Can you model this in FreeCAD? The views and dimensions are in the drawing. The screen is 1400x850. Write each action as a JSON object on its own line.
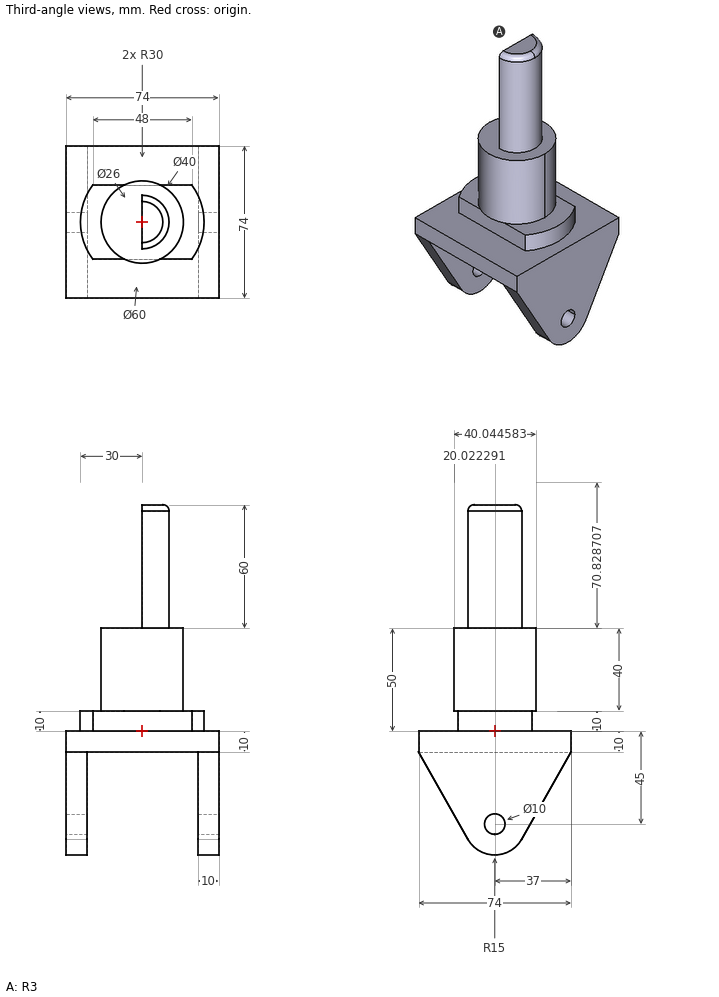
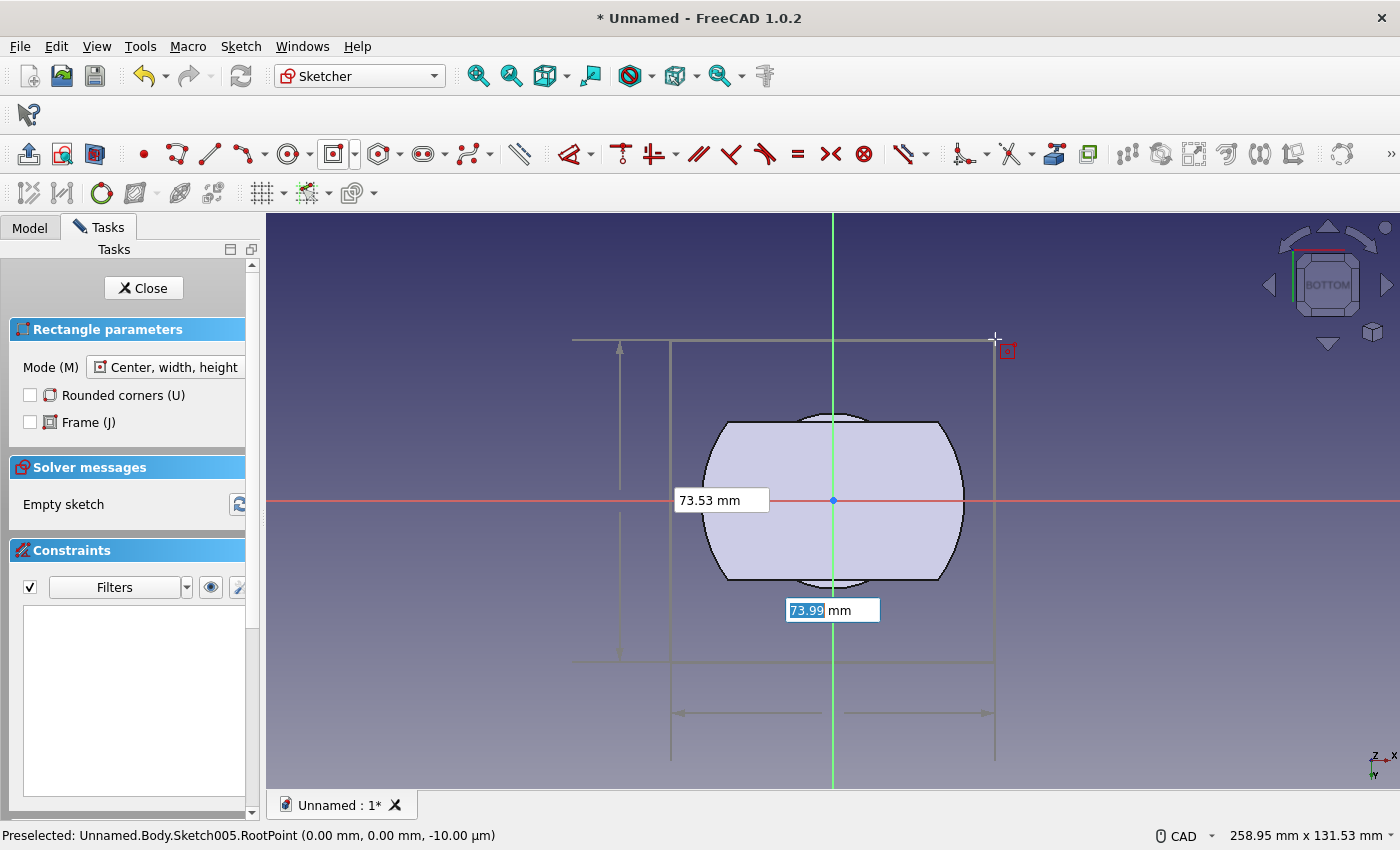
{"action": "type", "text": "74"}
{"action": "key", "text": "Tab"}
{"action": "type", "text": "74"}
{"action": "key", "text": "Return"}
{"action": "key", "text": "Escape"}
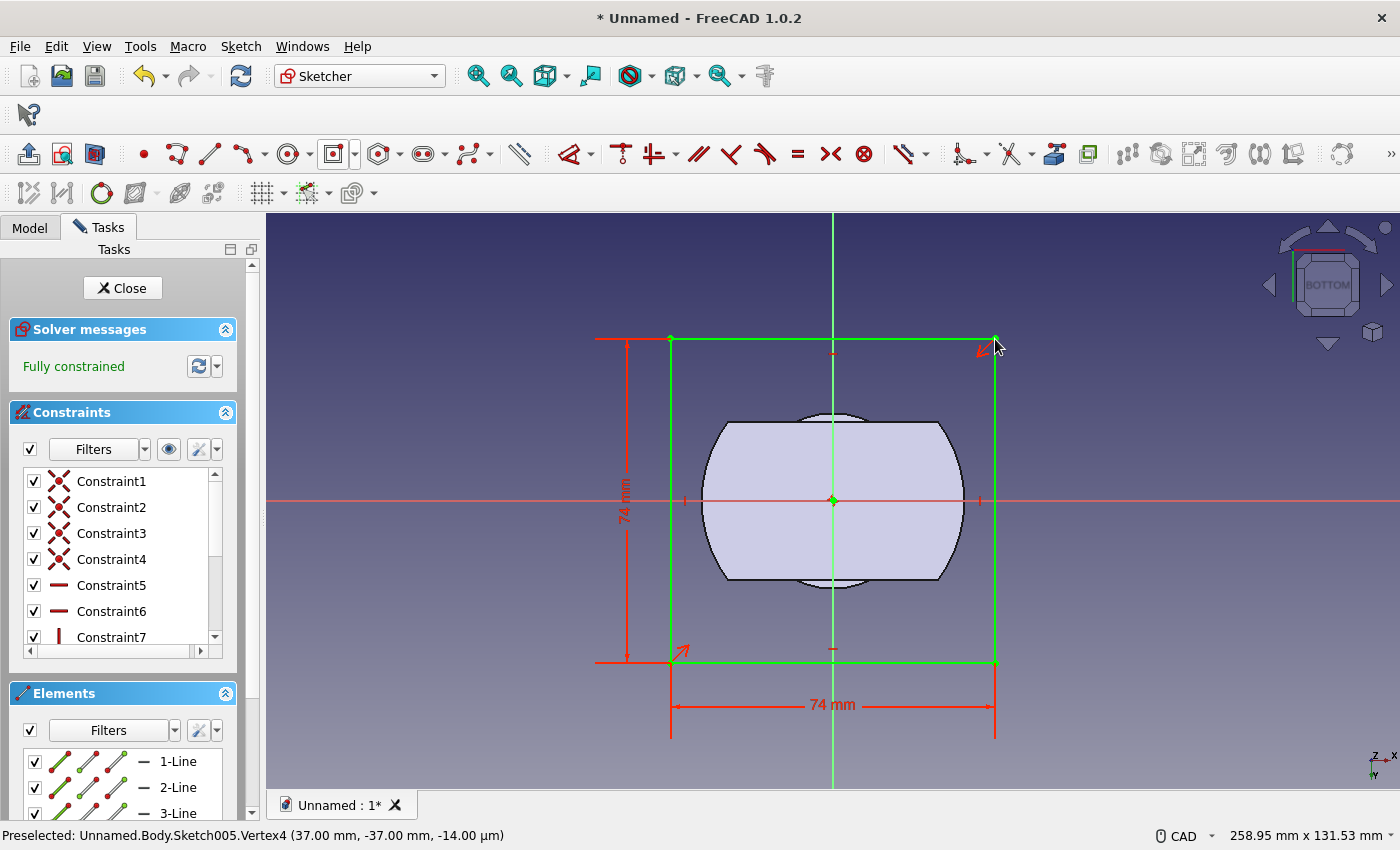
{"action": "left_click", "coordinate": [123, 288]}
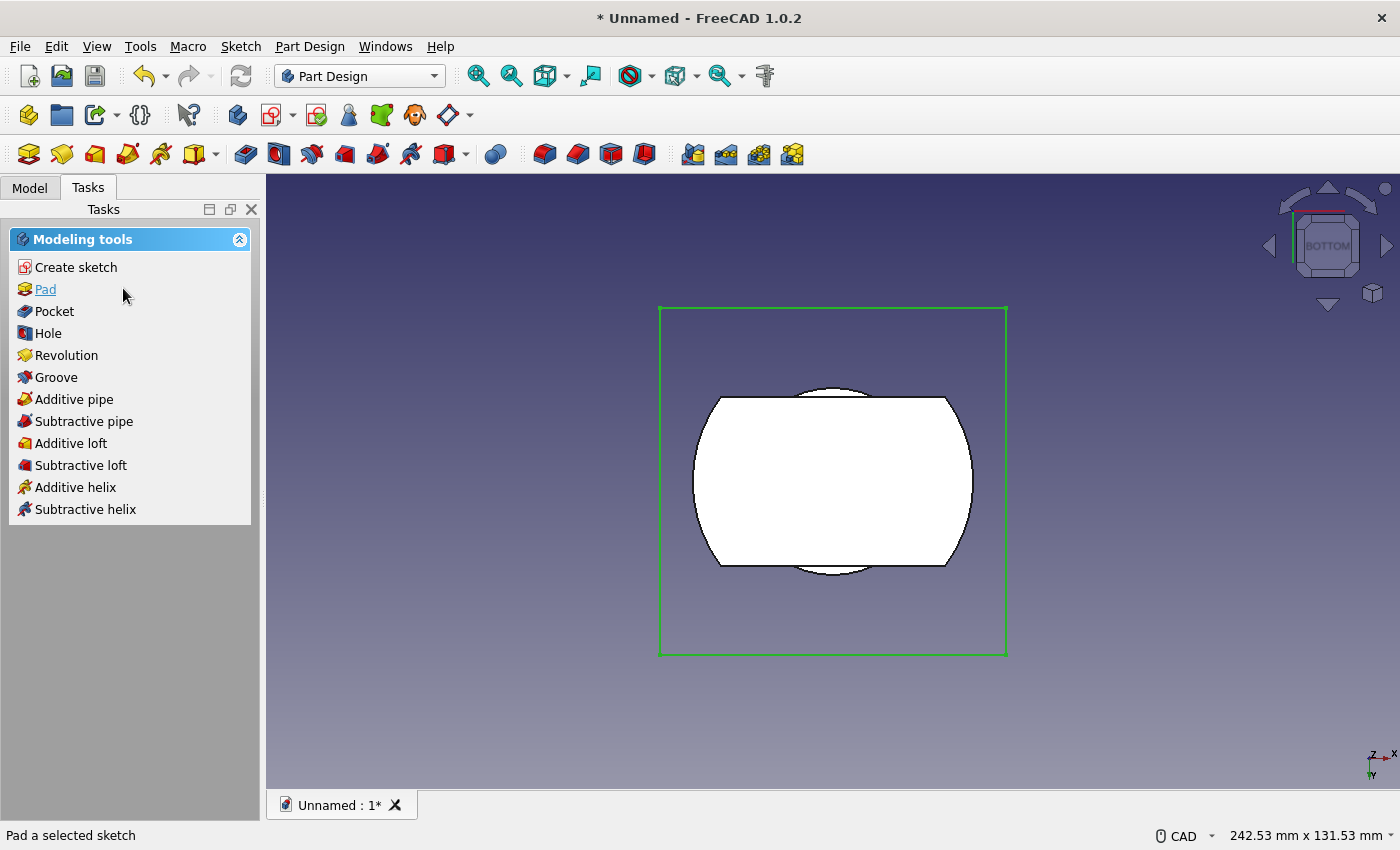
{"action": "left_click", "coordinate": [29, 154]}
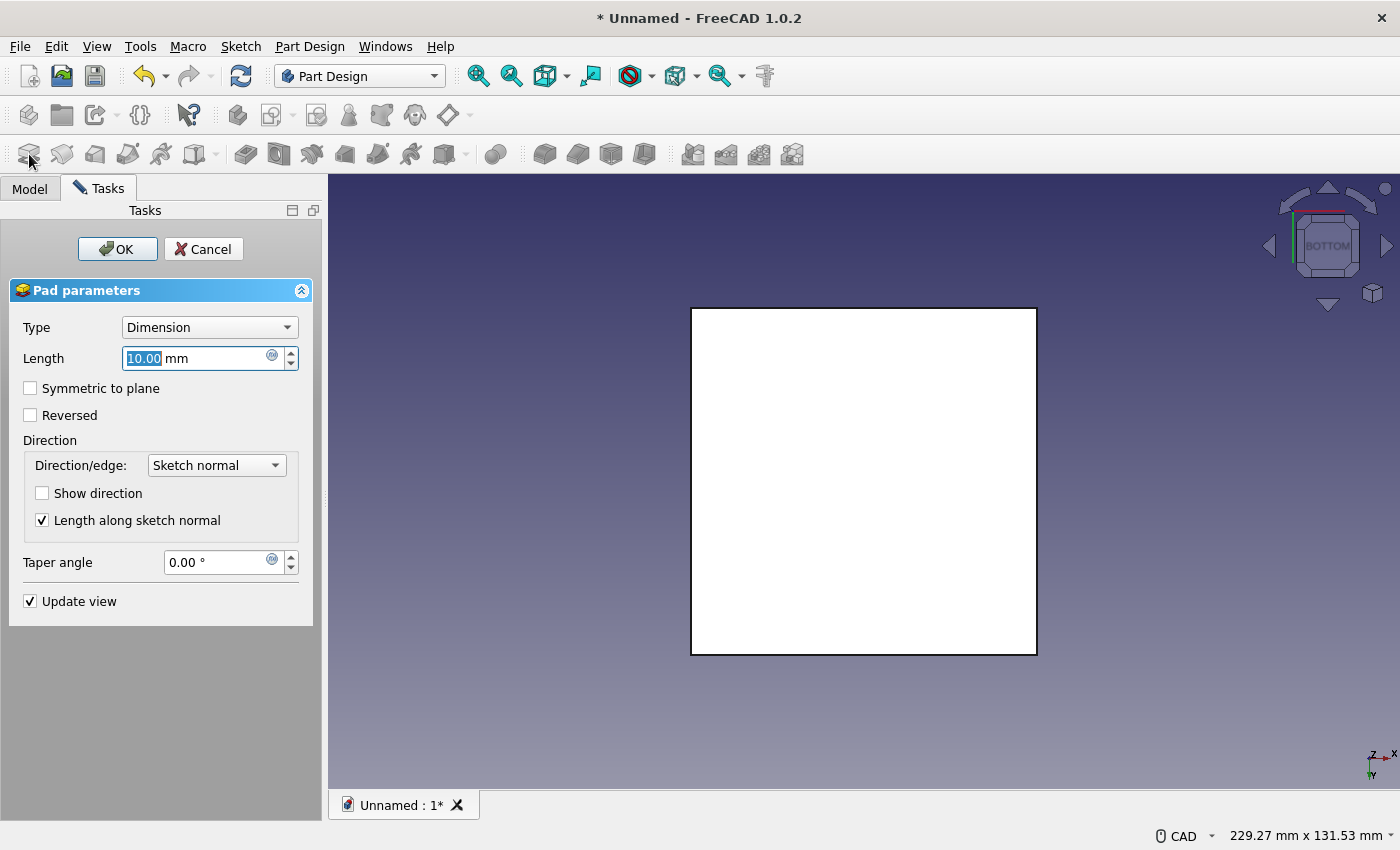
{"action": "type", "text": "10"}
{"action": "key", "text": "Tab"}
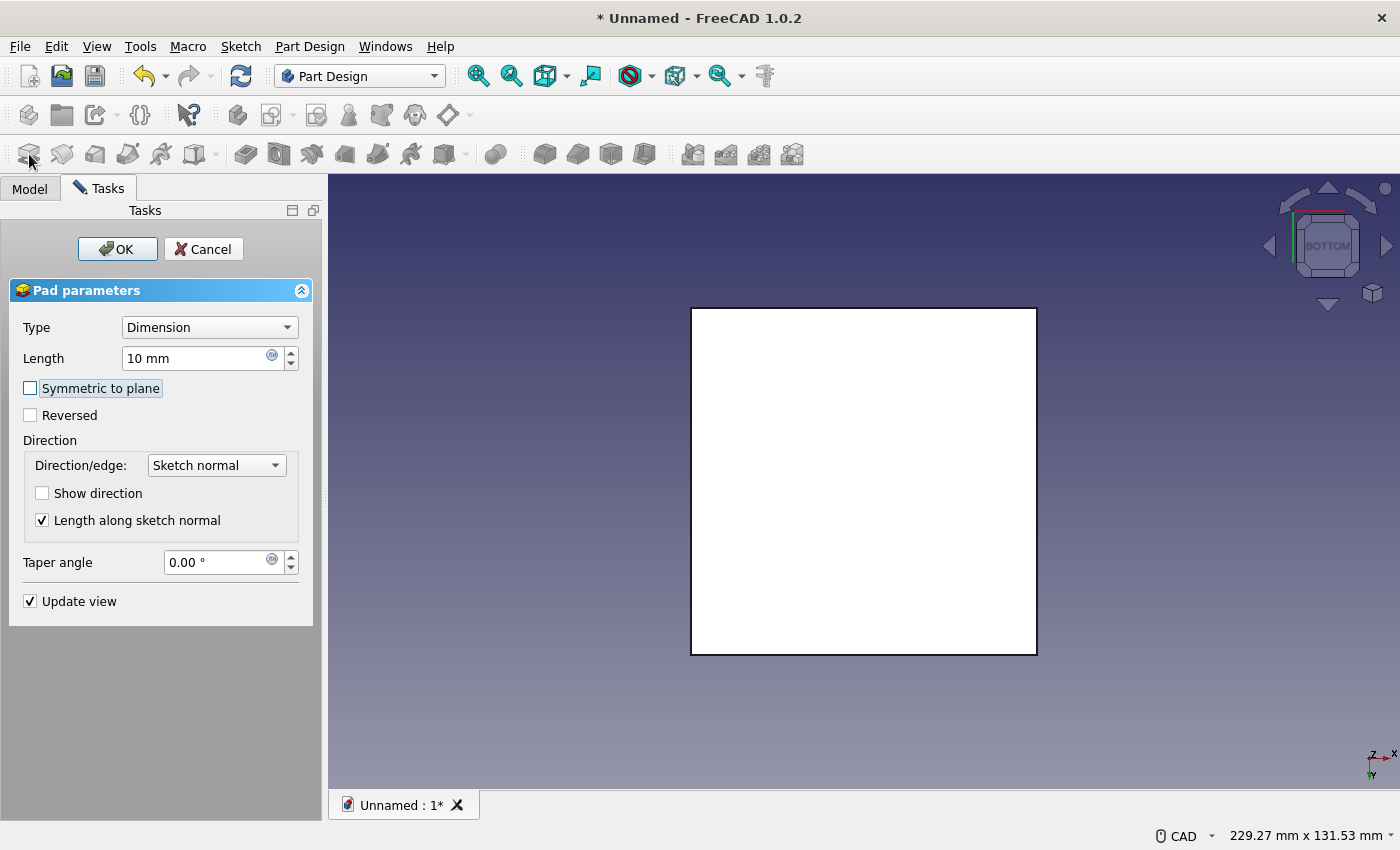
{"action": "left_click", "coordinate": [118, 249]}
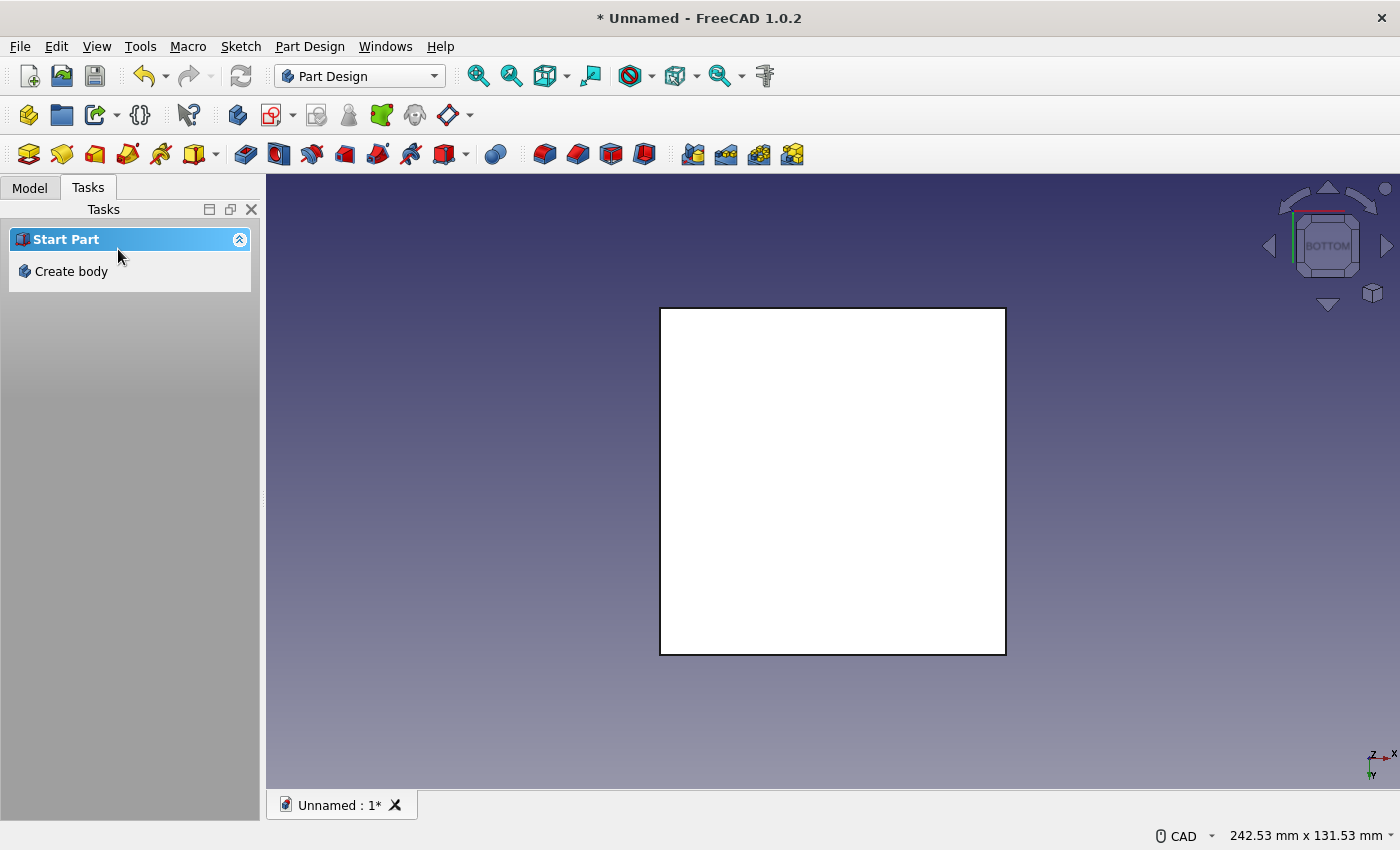
{"action": "key", "text": "0"}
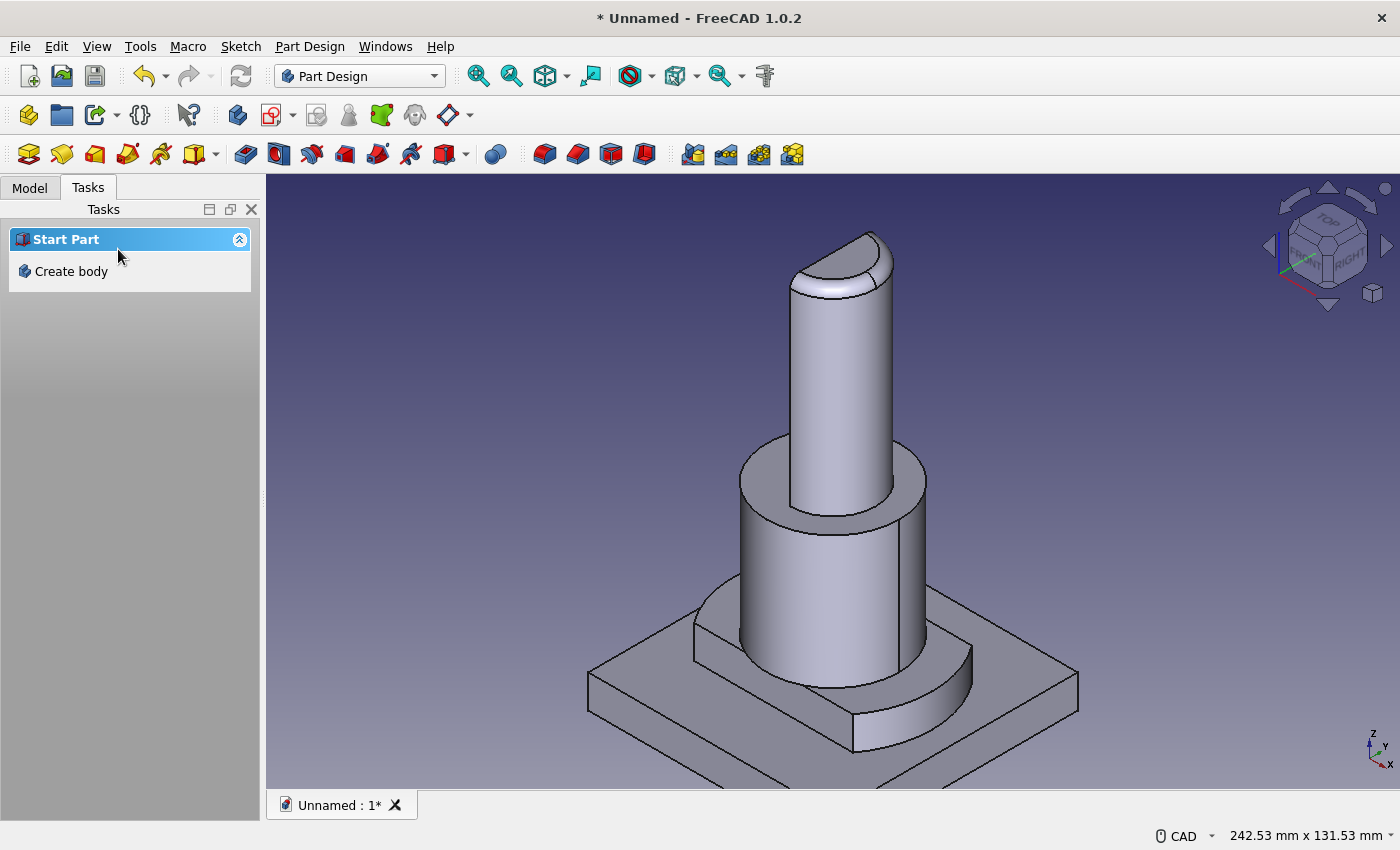
{"action": "left_click", "coordinate": [479, 76]}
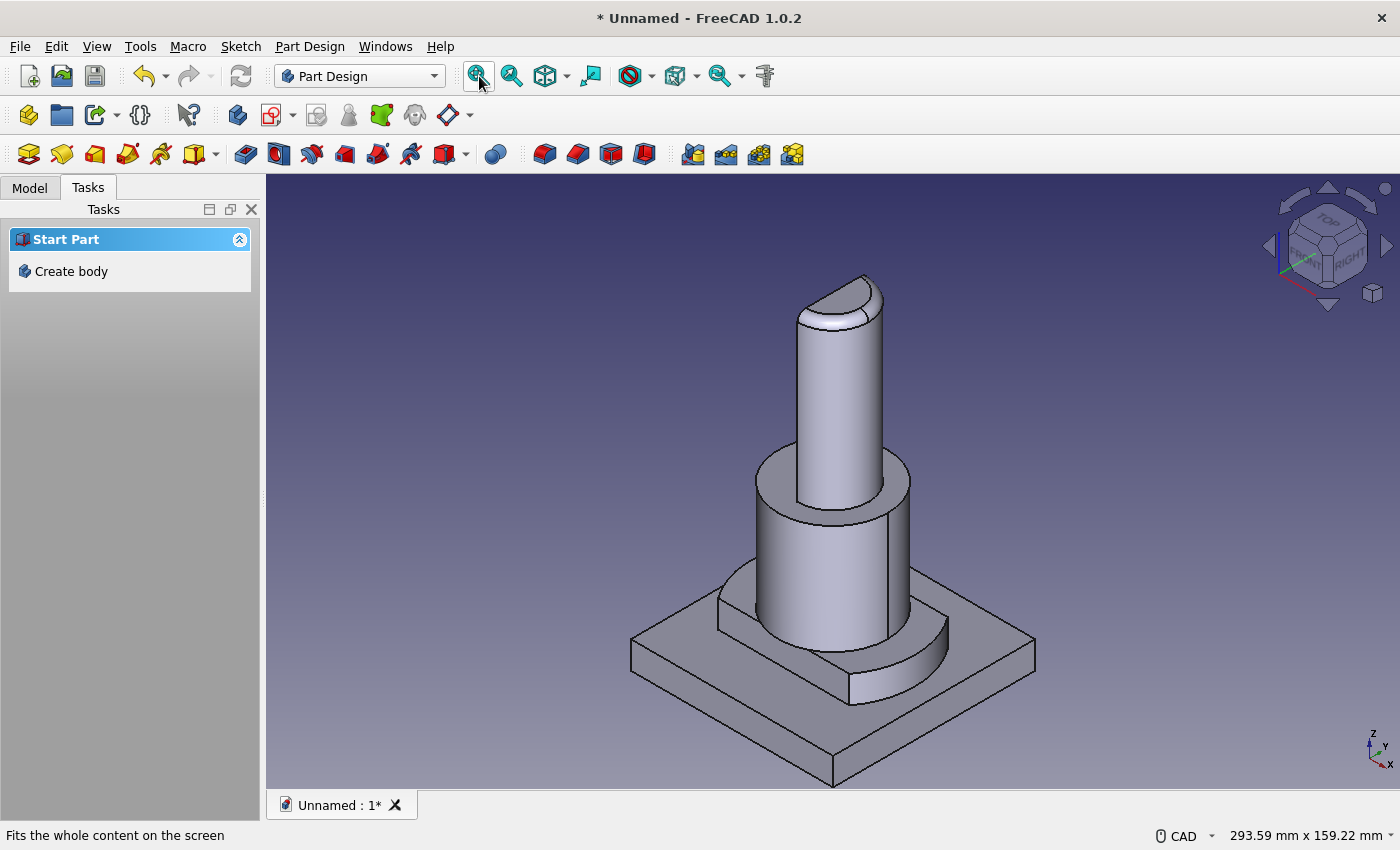
{"action": "left_click", "coordinate": [1021, 662]}